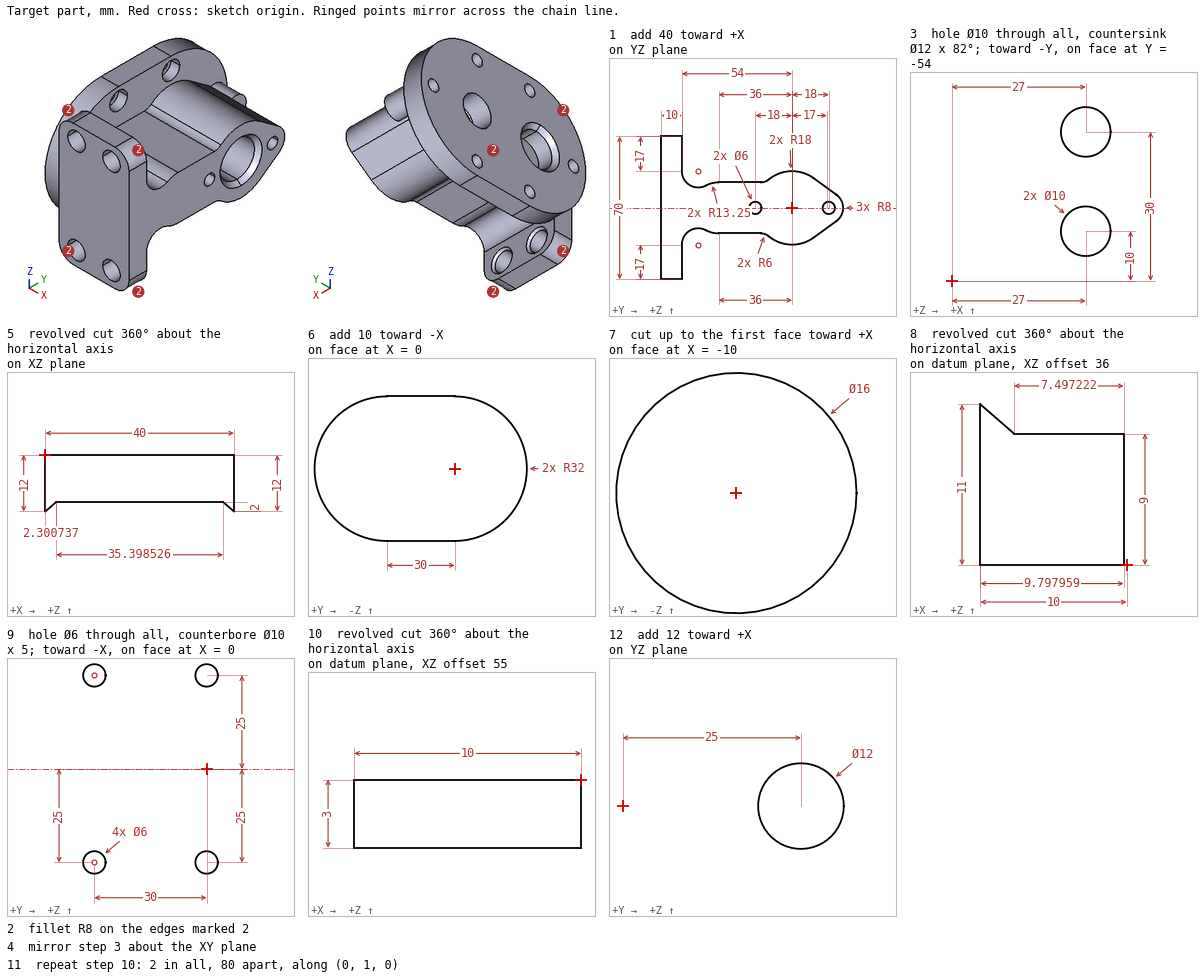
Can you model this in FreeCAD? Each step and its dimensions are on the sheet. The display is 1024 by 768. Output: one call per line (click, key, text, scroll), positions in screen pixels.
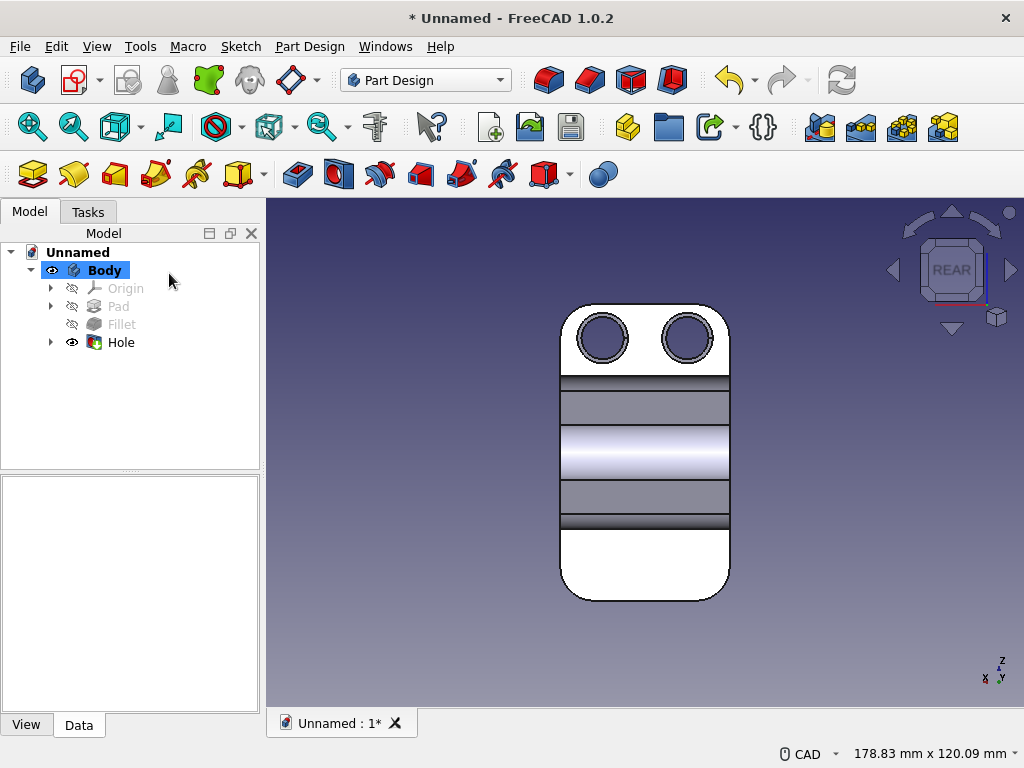
click(117, 342)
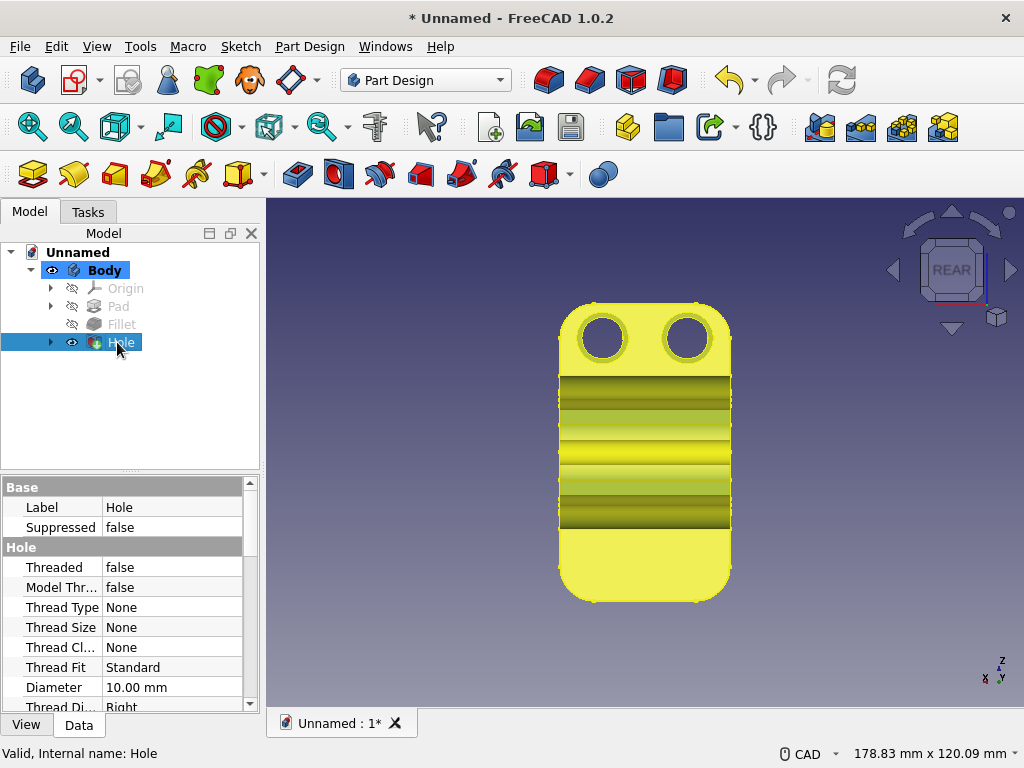
click(820, 128)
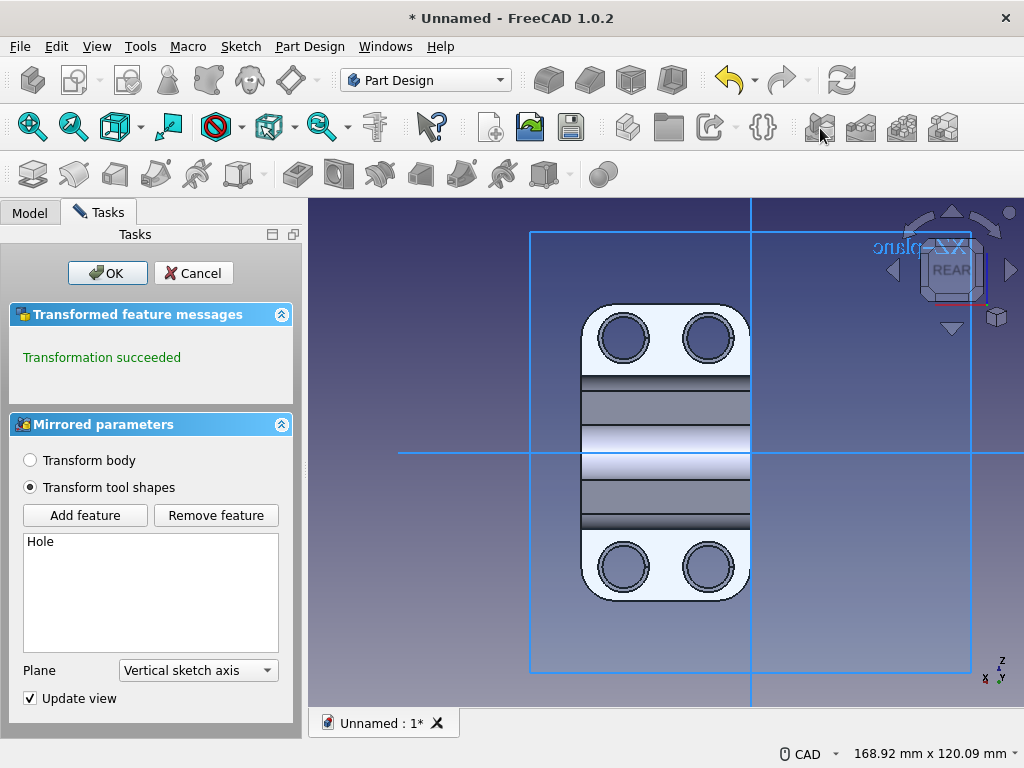
click(199, 670)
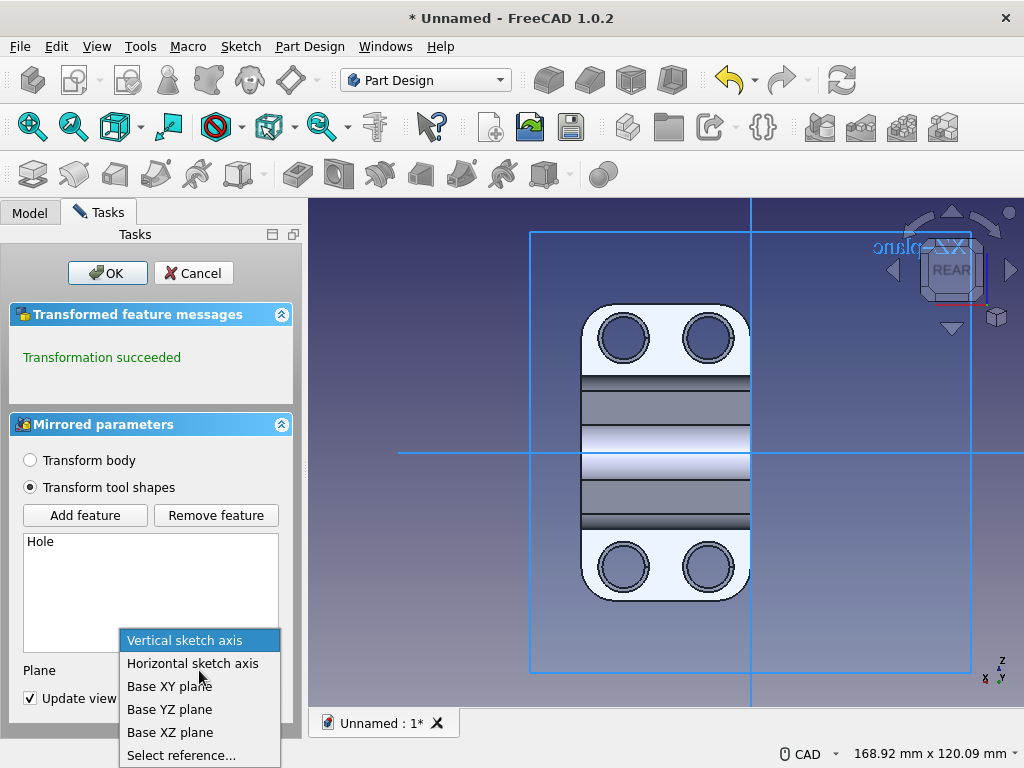
click(198, 686)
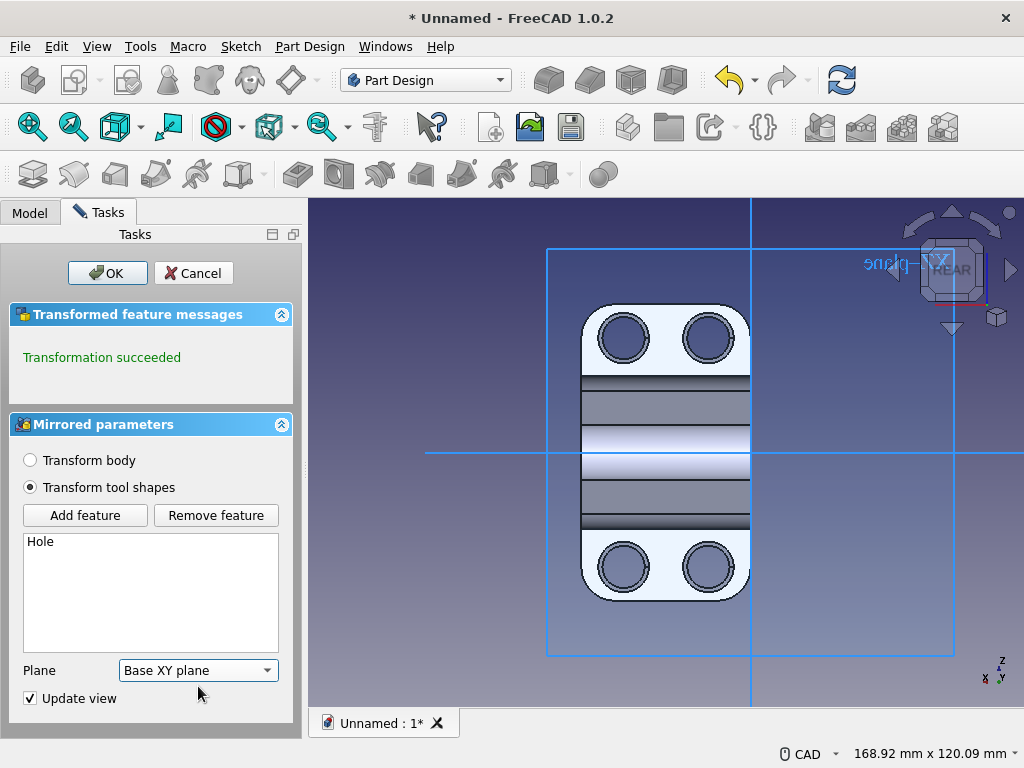
click(108, 273)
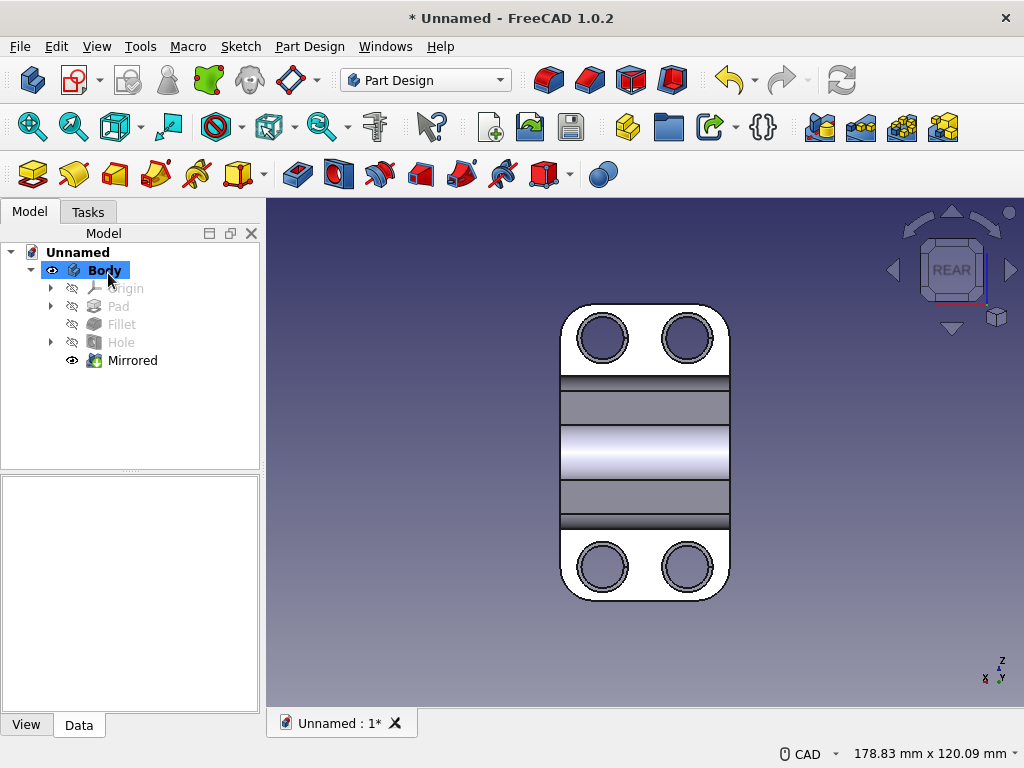
click(74, 80)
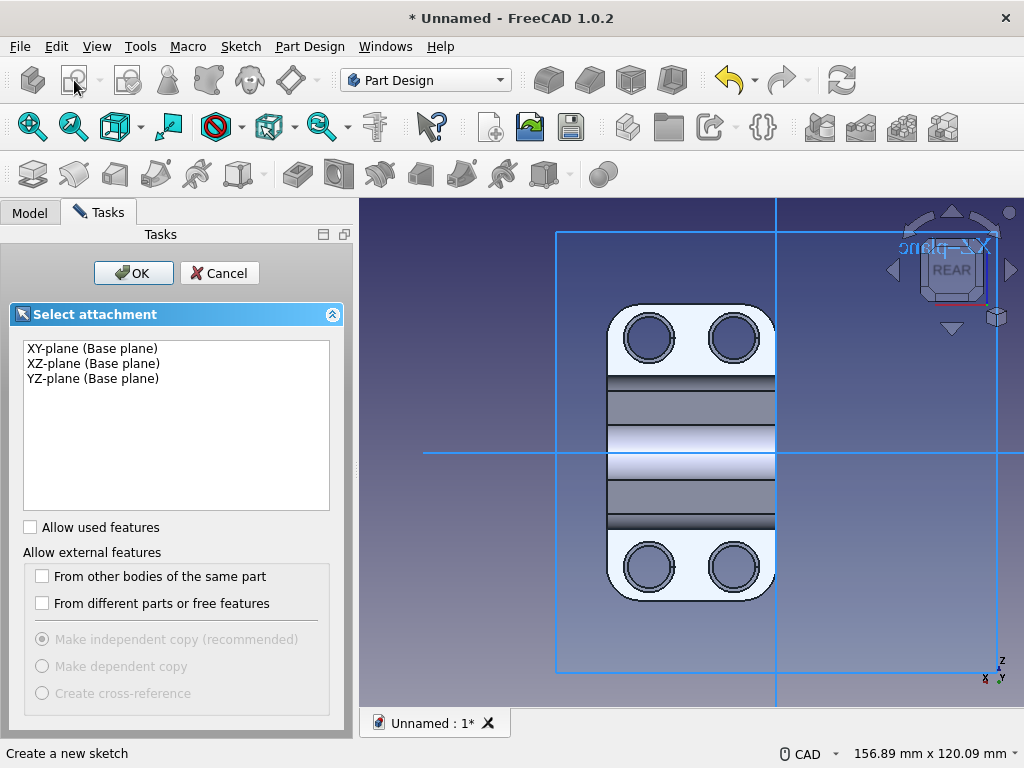
click(84, 364)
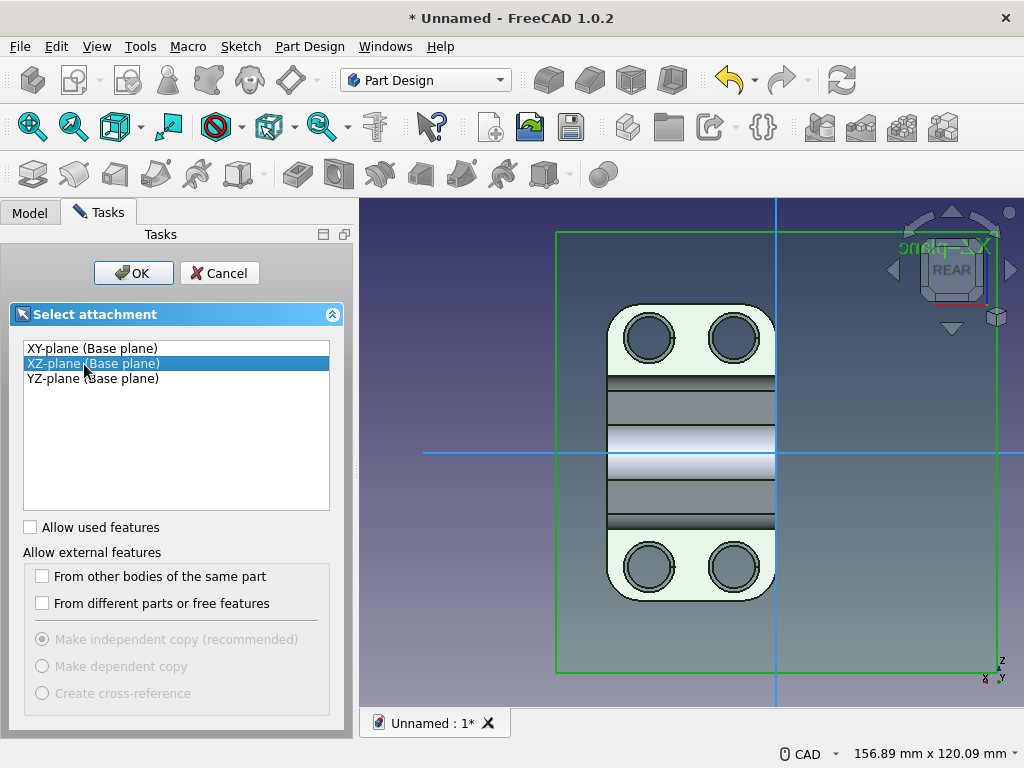
click(134, 273)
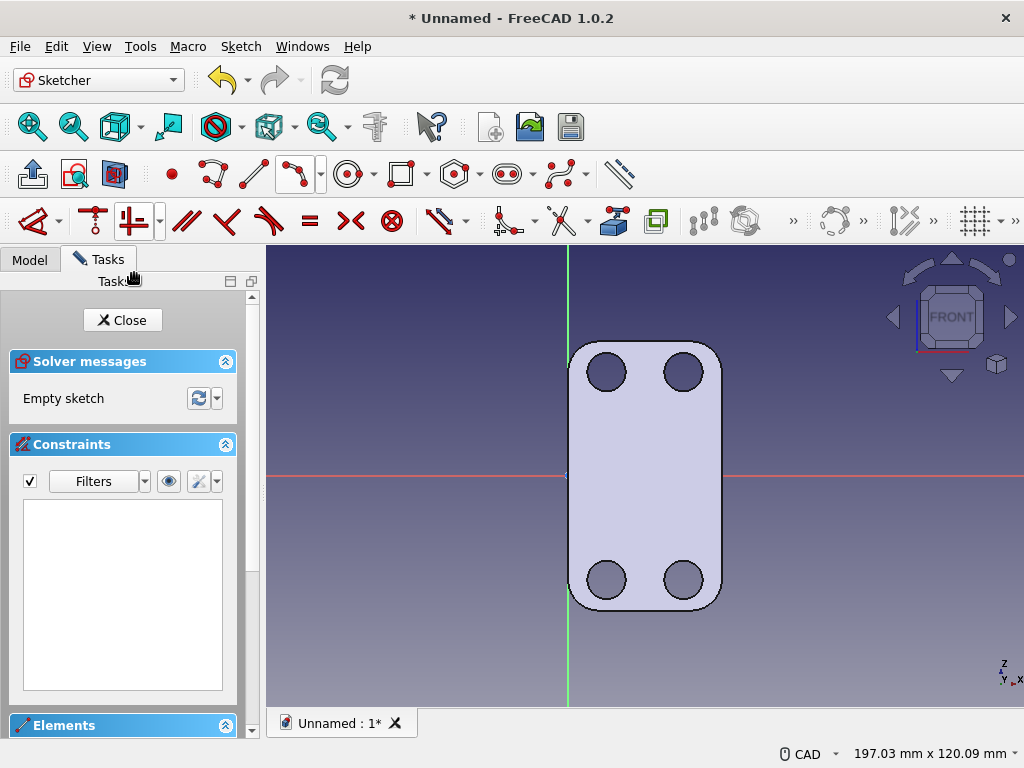
click(115, 174)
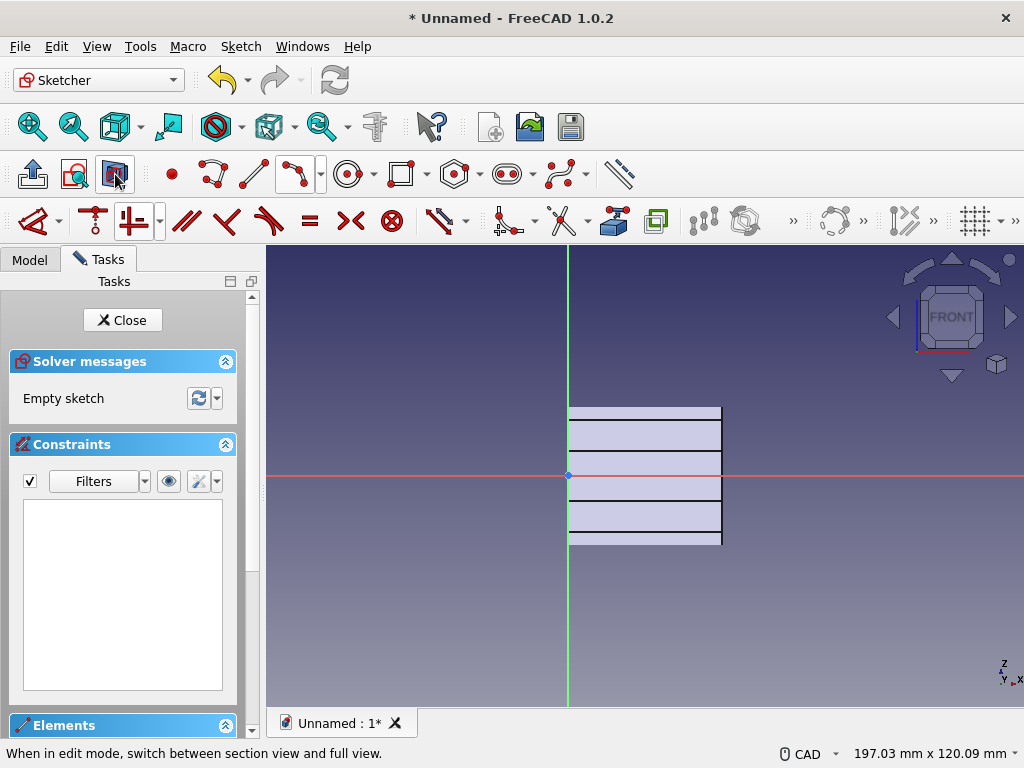
scroll(685, 513, up, 5)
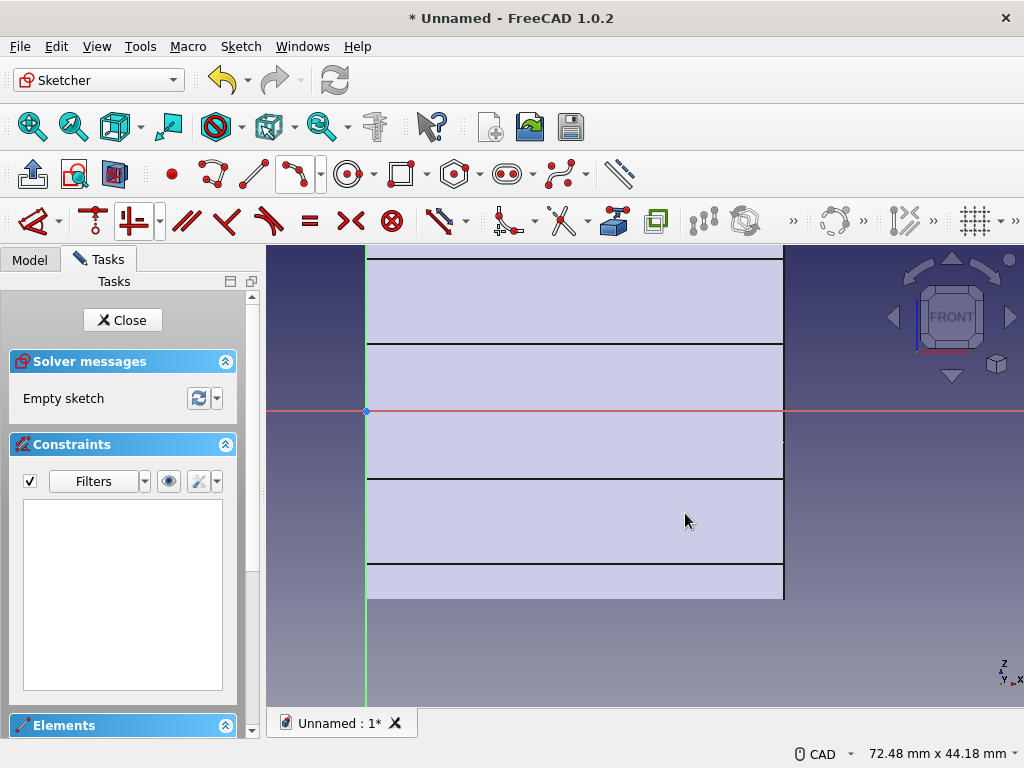
click(213, 174)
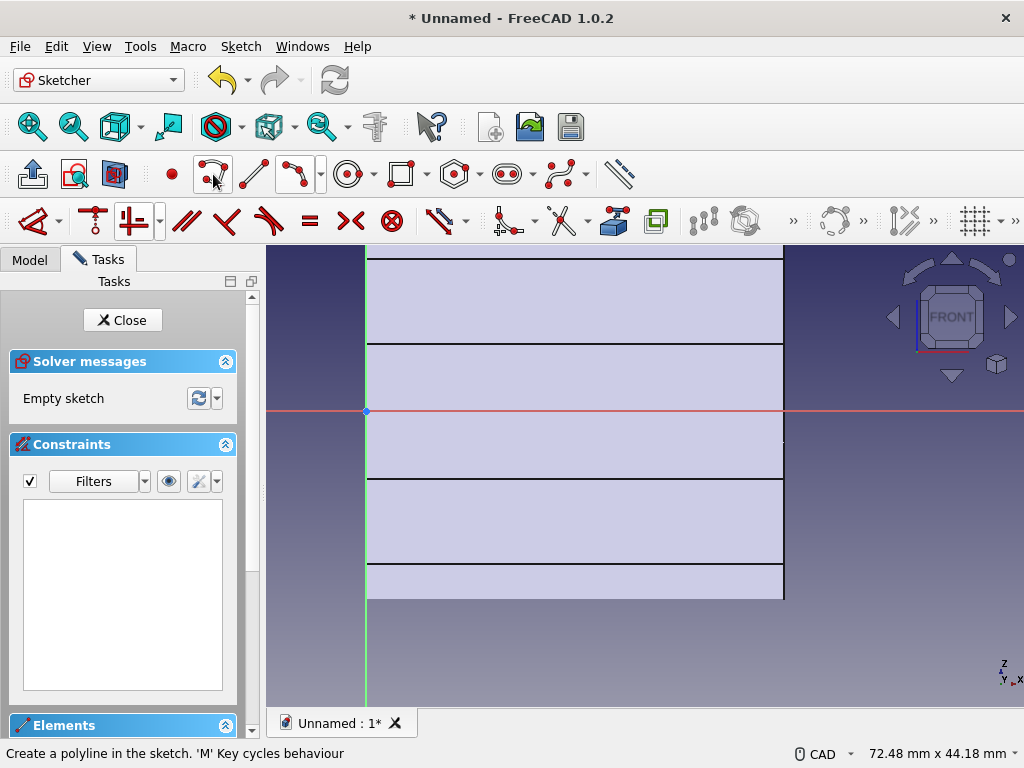
click(366, 411)
click(784, 420)
click(784, 537)
click(760, 516)
click(390, 516)
click(375, 537)
click(366, 411)
key(Escape)
key(Escape)